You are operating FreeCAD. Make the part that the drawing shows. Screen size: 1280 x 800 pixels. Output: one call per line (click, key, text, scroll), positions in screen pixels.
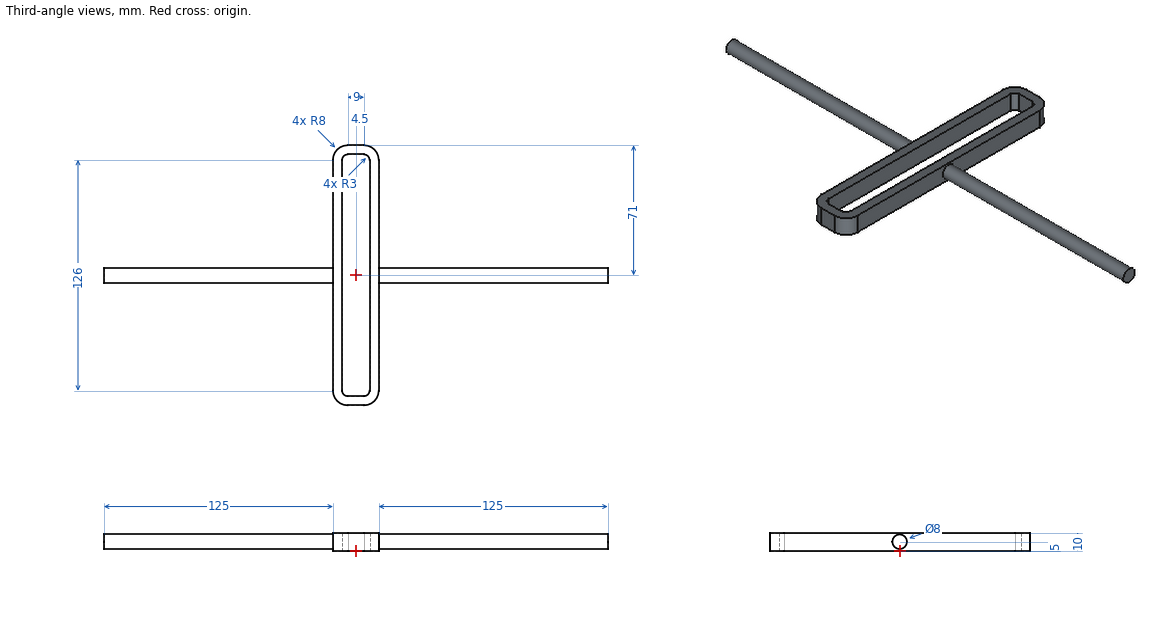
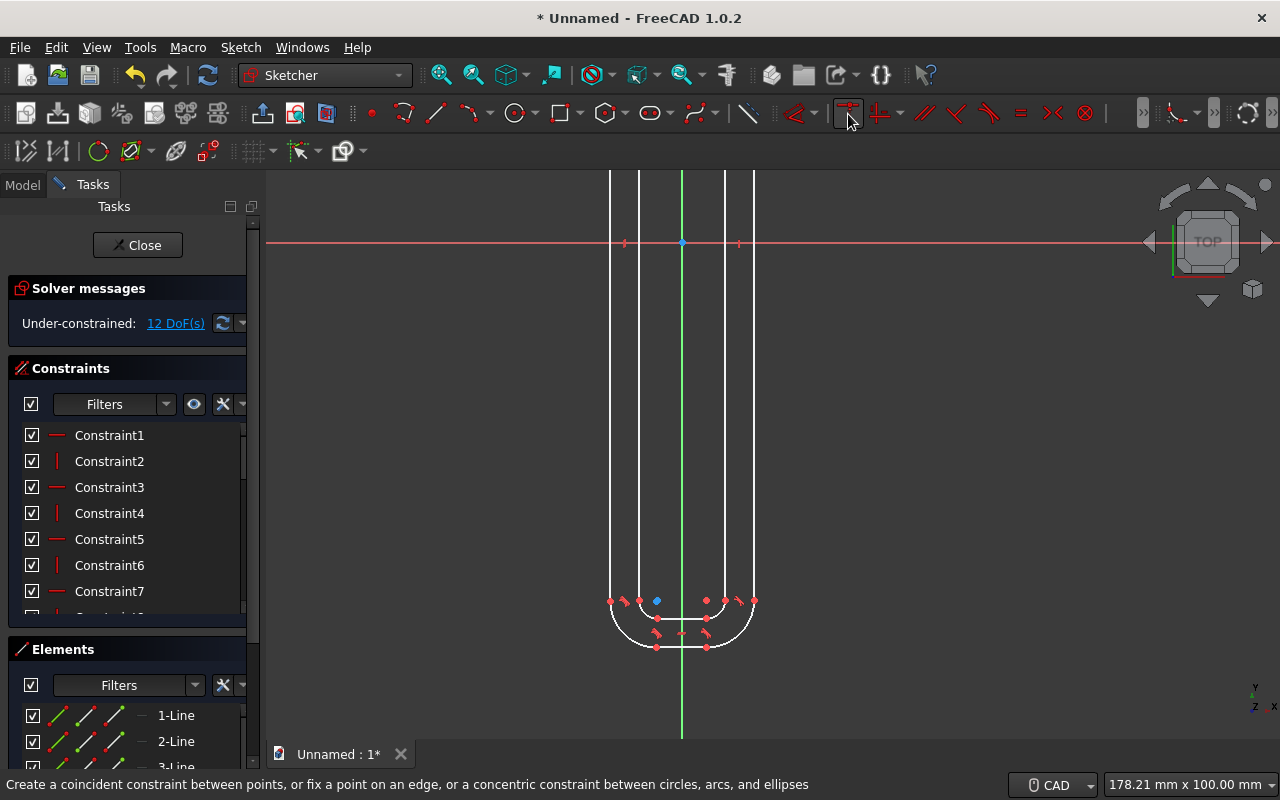
click(615, 622)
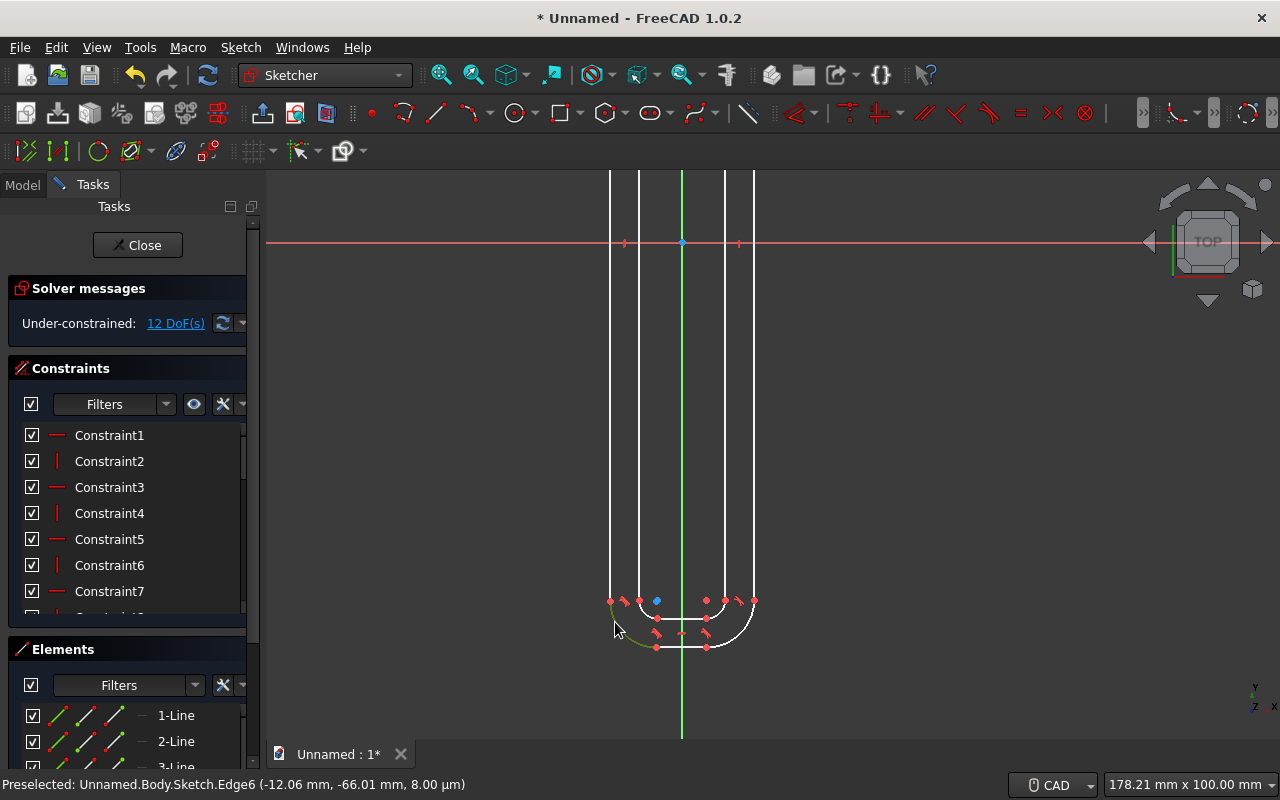
click(645, 613)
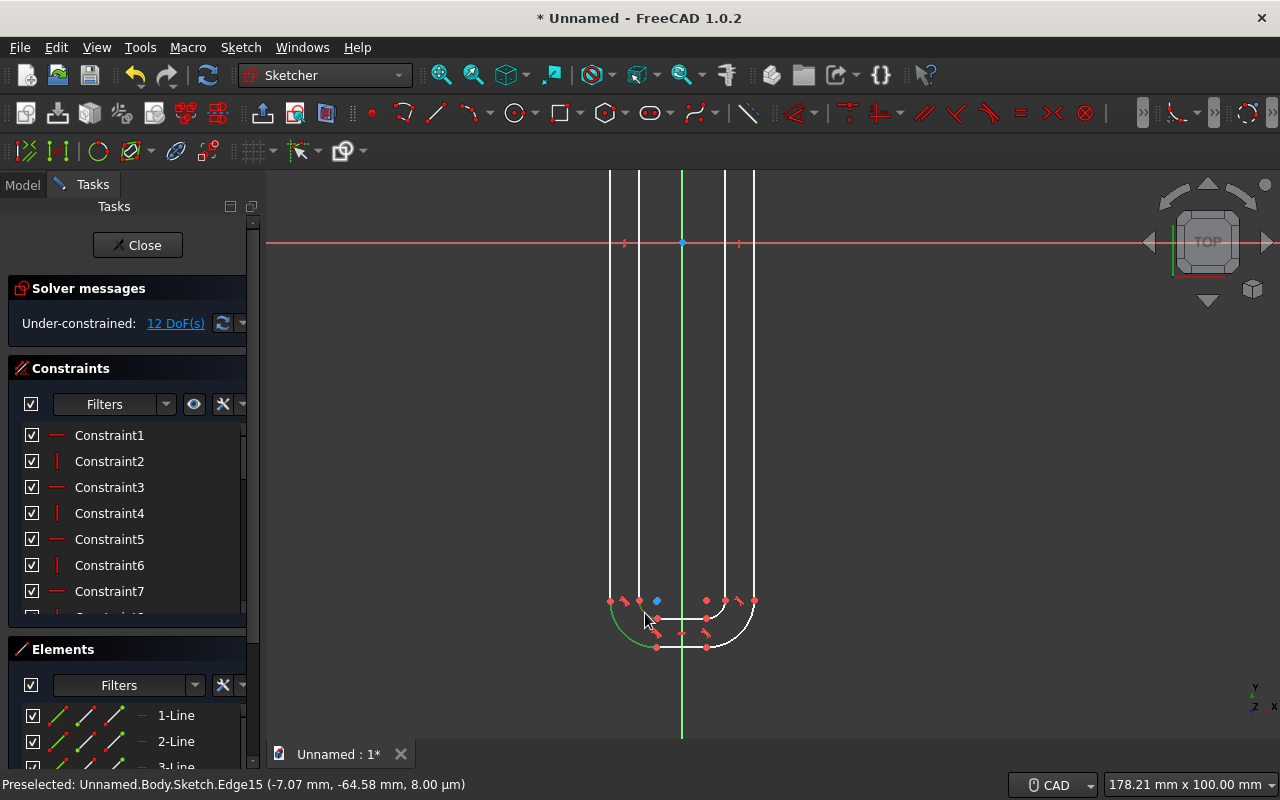
click(848, 114)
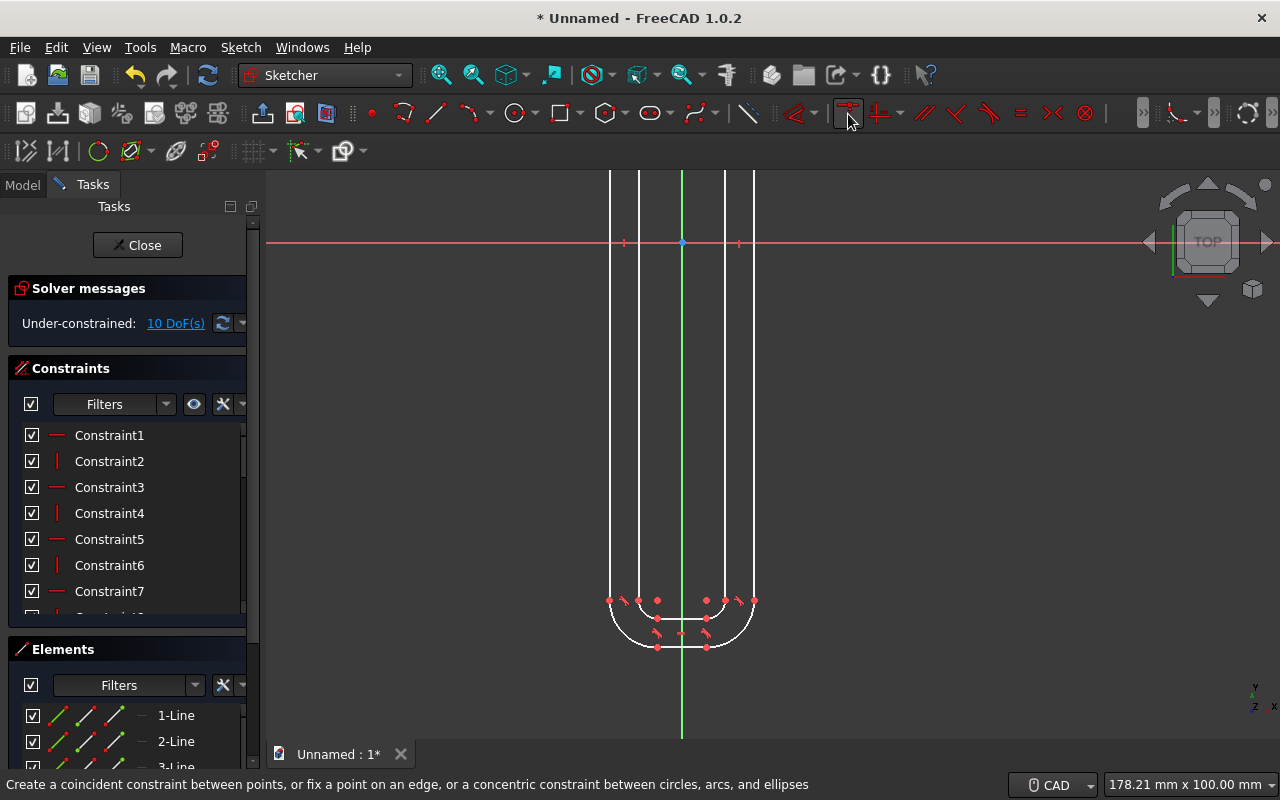
scroll(723, 627, down, 4)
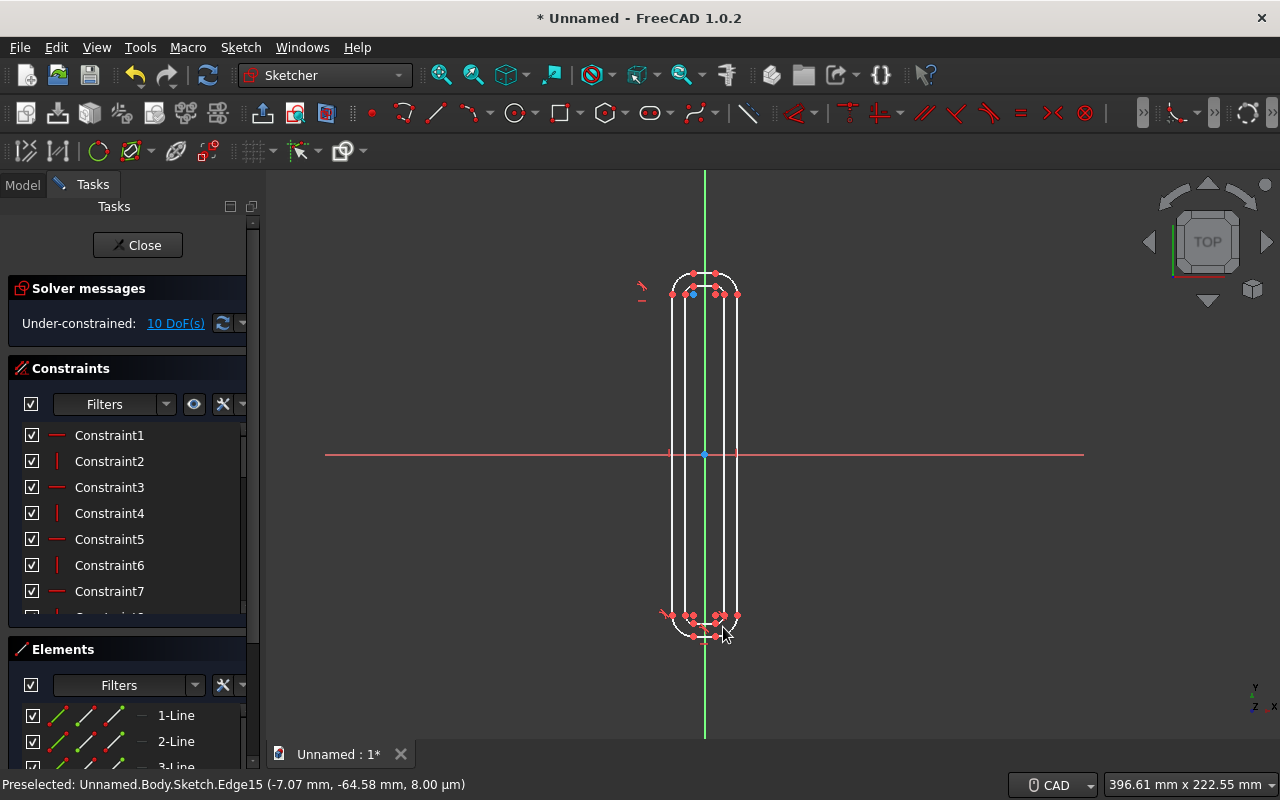
scroll(684, 276, up, 2)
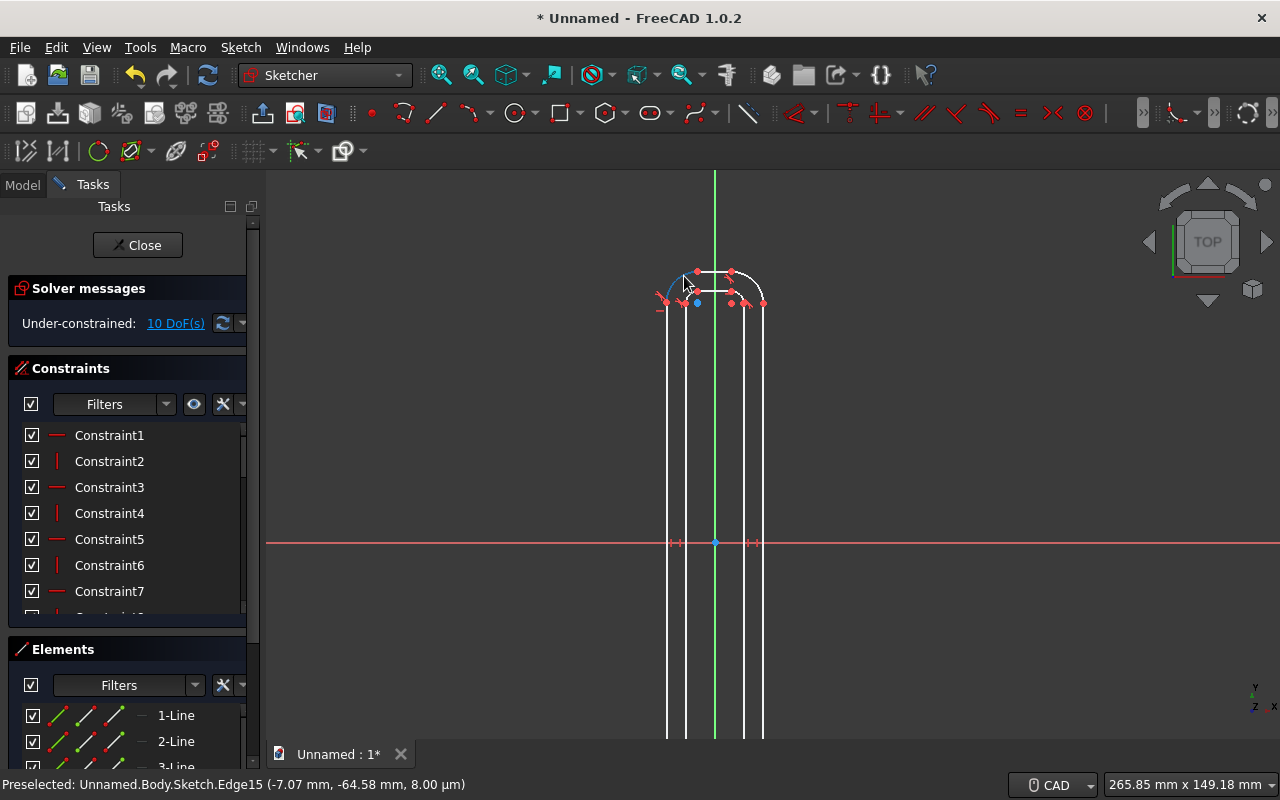
click(683, 275)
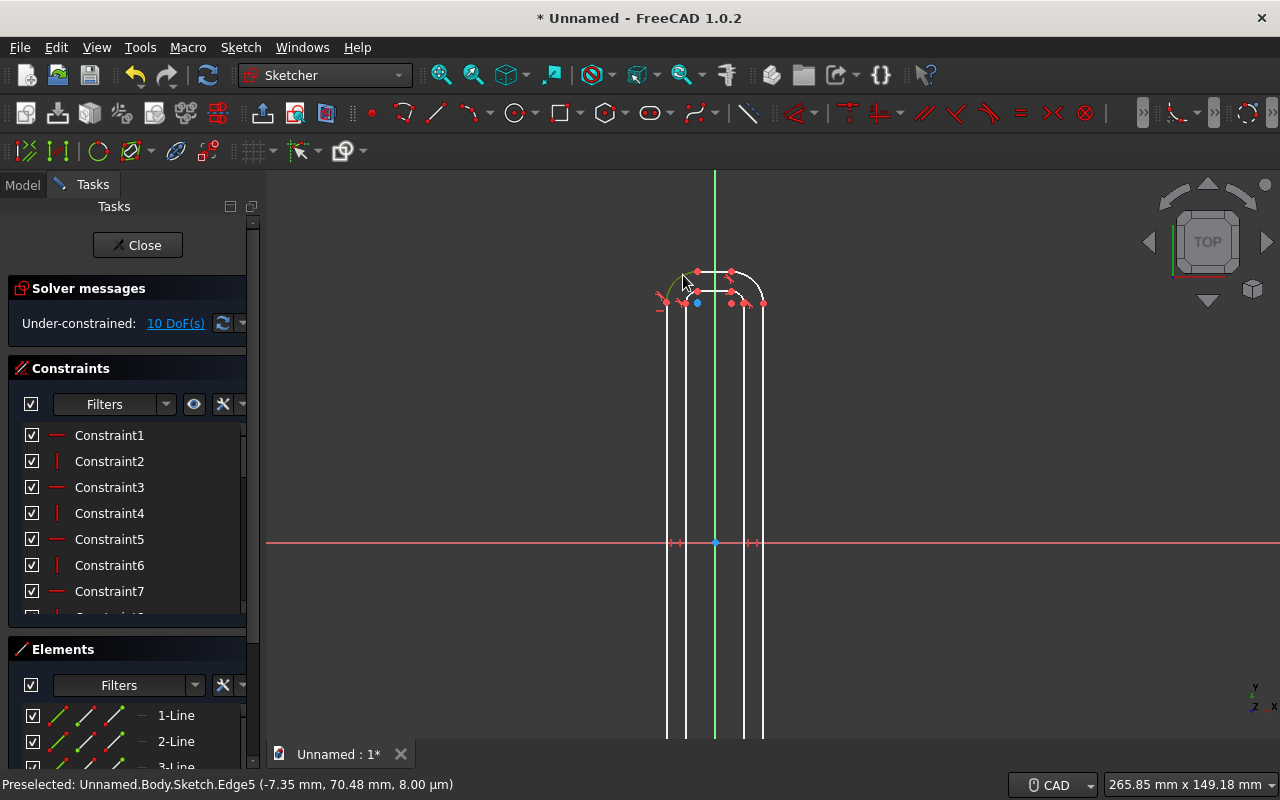
scroll(683, 275, down, 2)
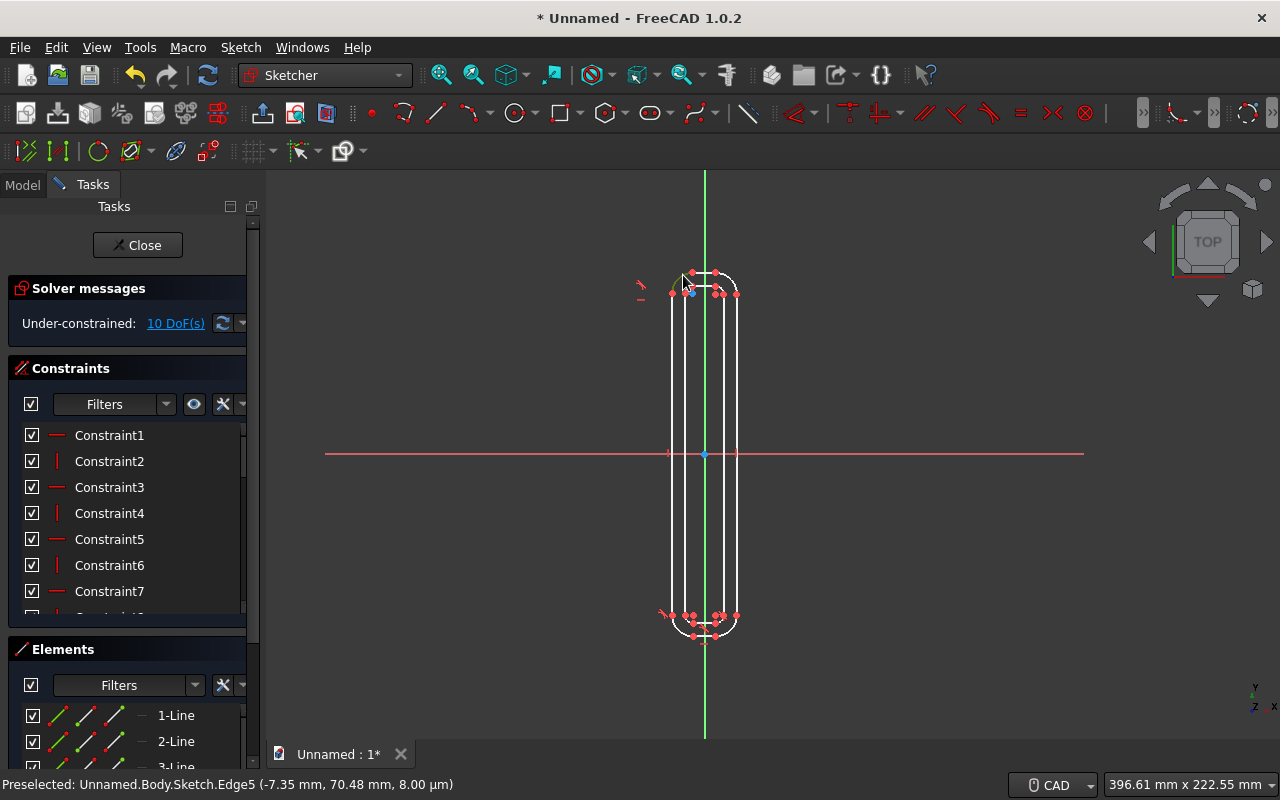
scroll(674, 625, up, 2)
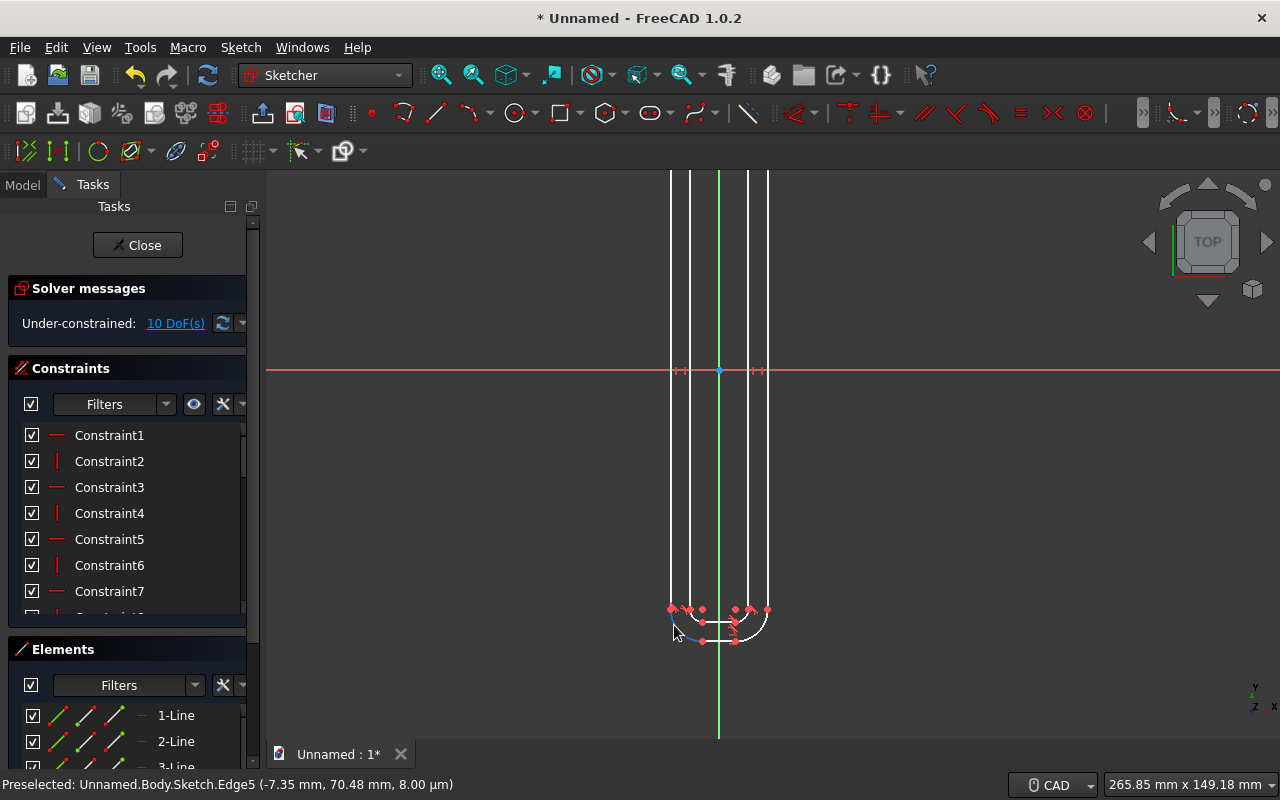
click(674, 624)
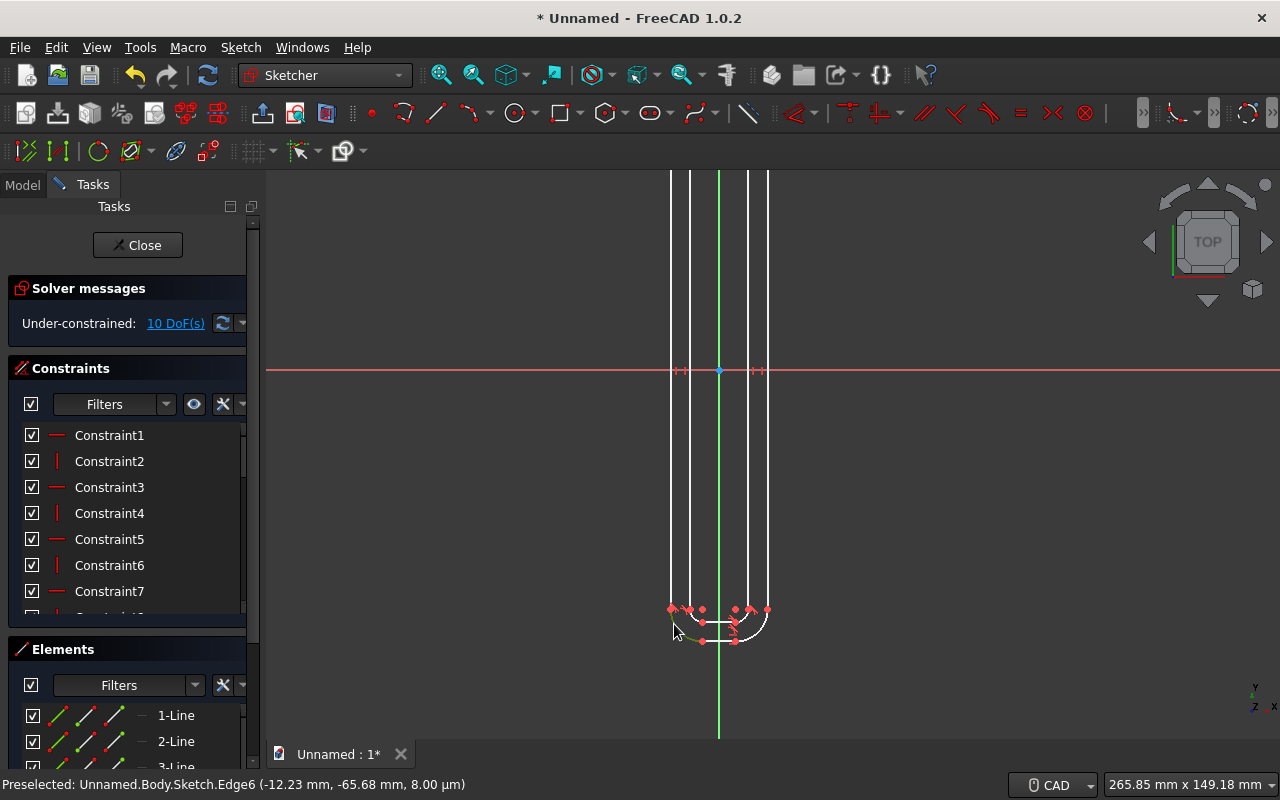
click(750, 638)